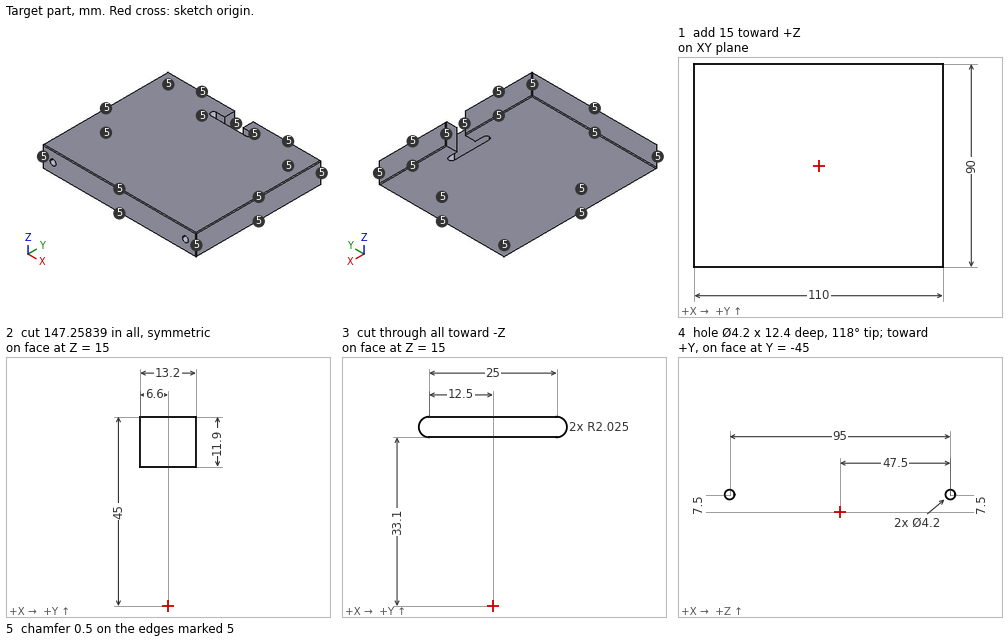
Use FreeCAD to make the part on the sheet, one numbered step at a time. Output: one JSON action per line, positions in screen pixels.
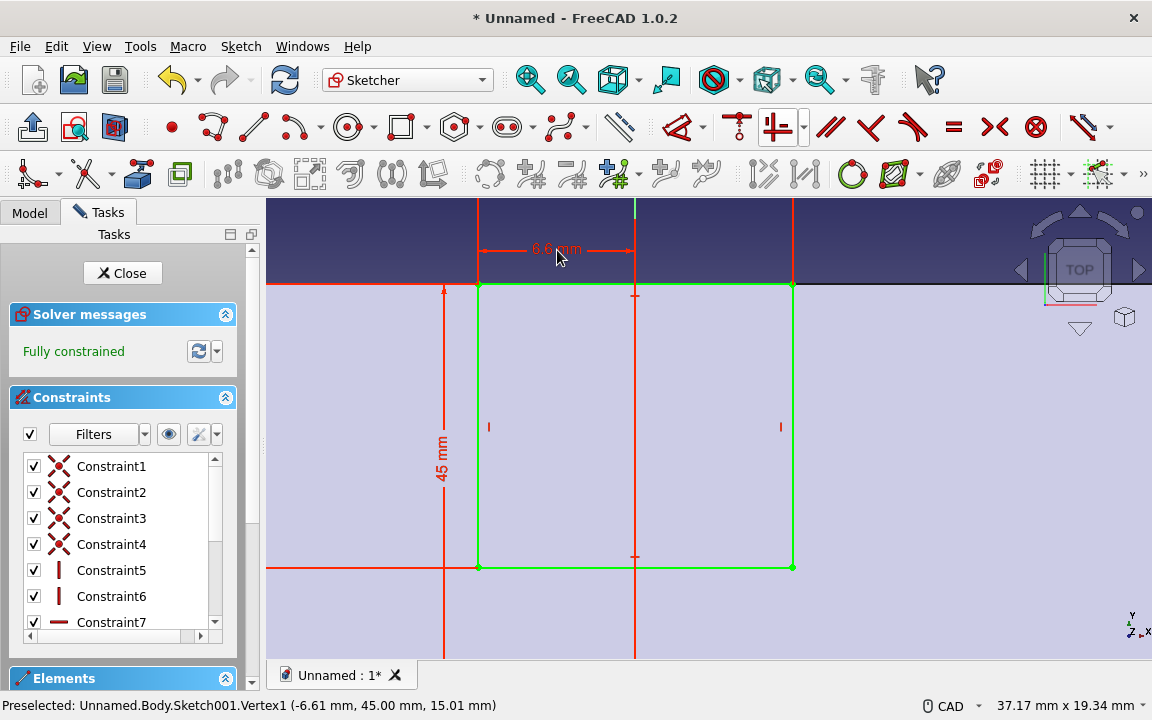
{"action": "left_click", "coordinate": [123, 273]}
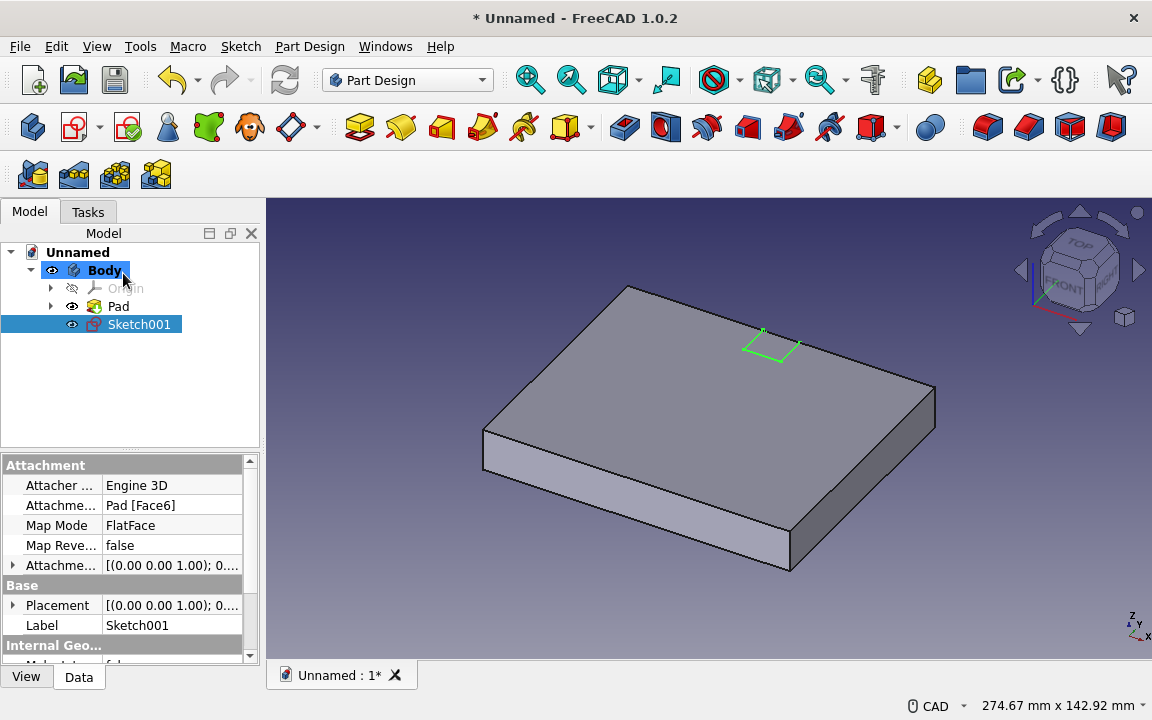
{"action": "left_click", "coordinate": [625, 128]}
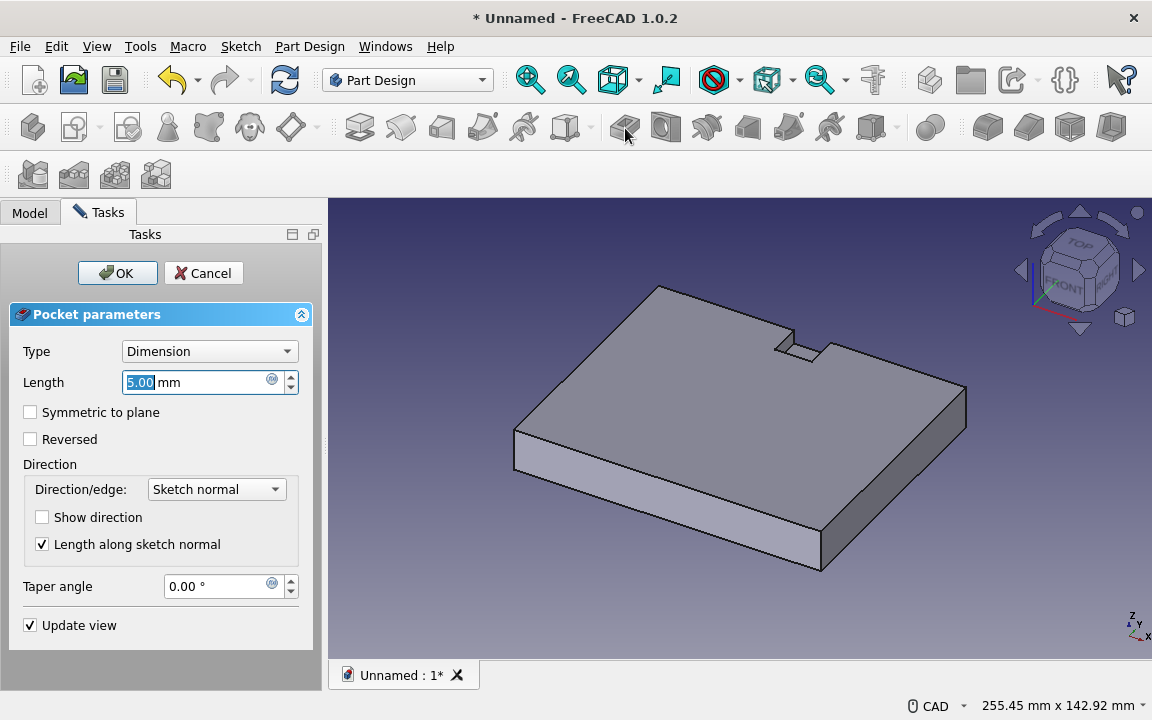
{"action": "type", "text": "147.25839"}
{"action": "key", "text": "Tab"}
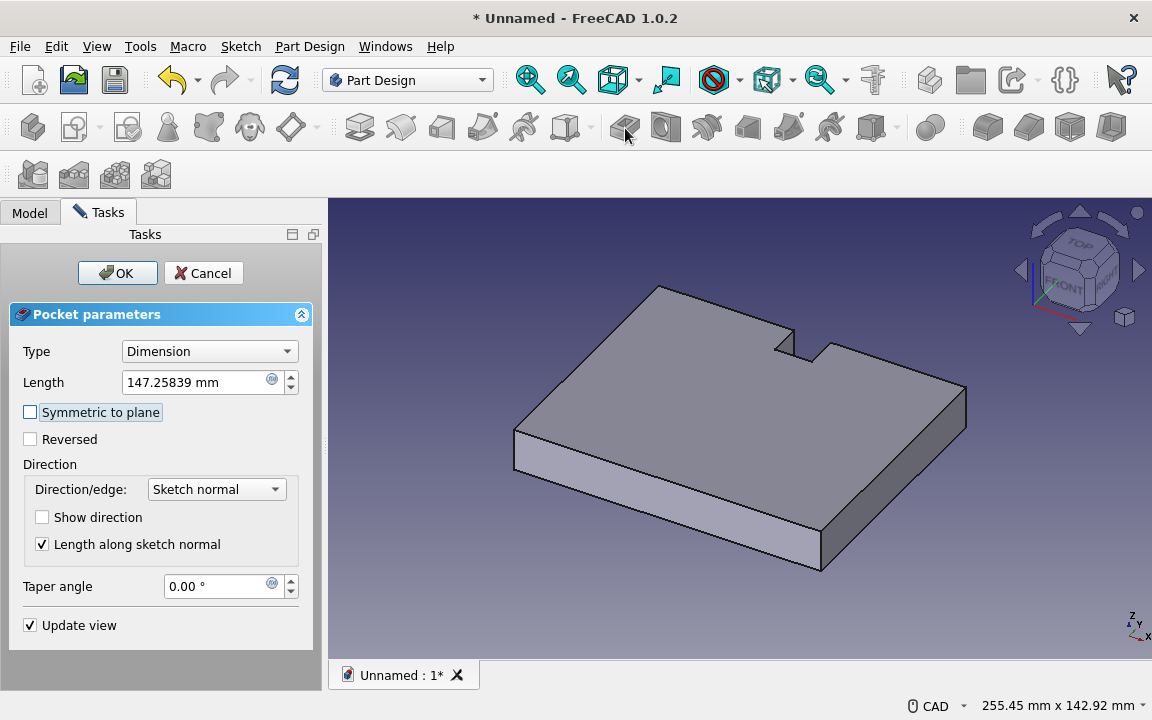
{"action": "left_click", "coordinate": [31, 412]}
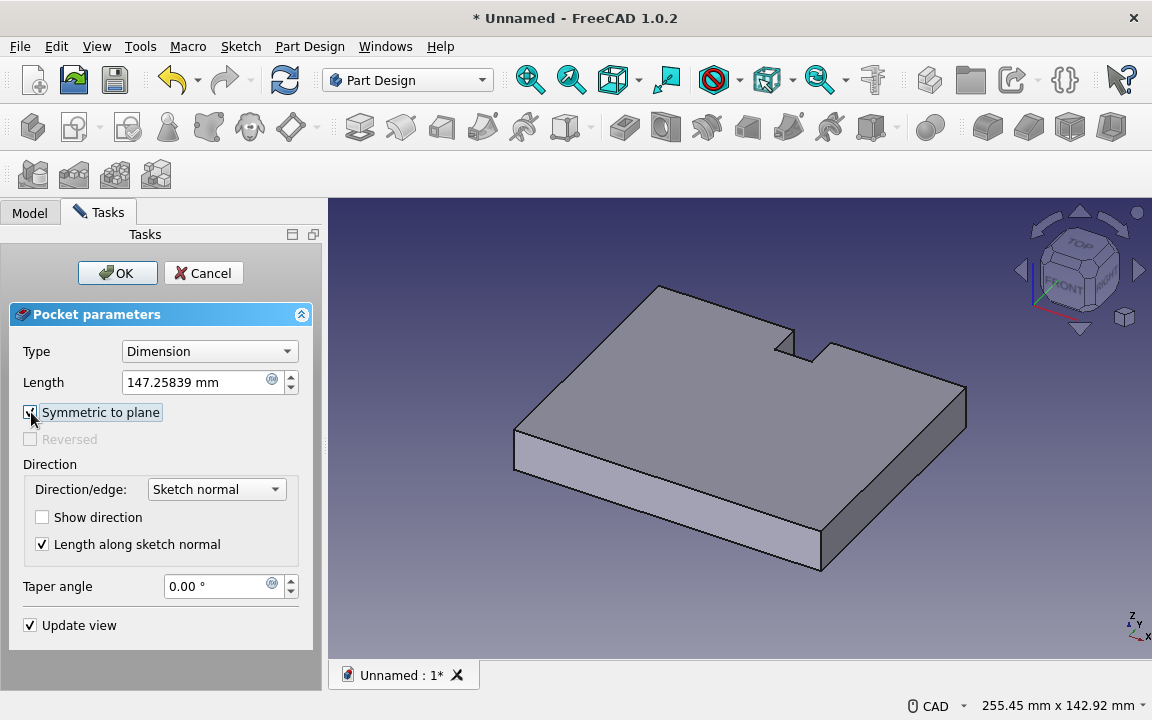
{"action": "left_click", "coordinate": [118, 273]}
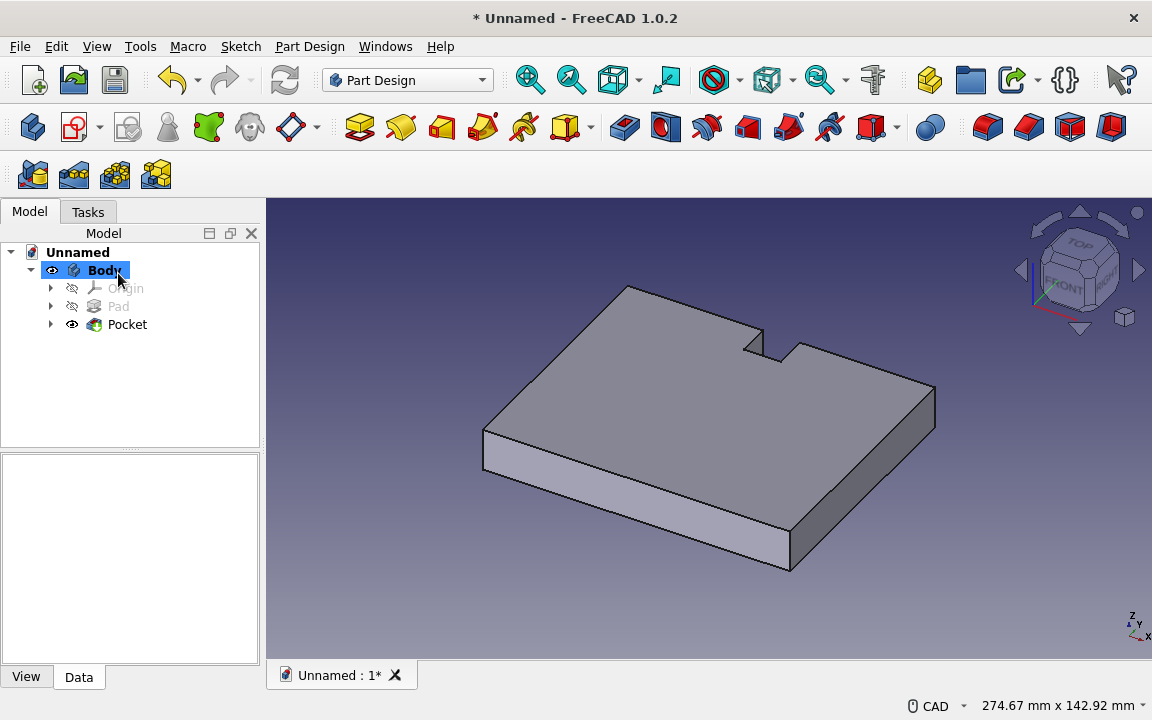
{"action": "left_click", "coordinate": [665, 393]}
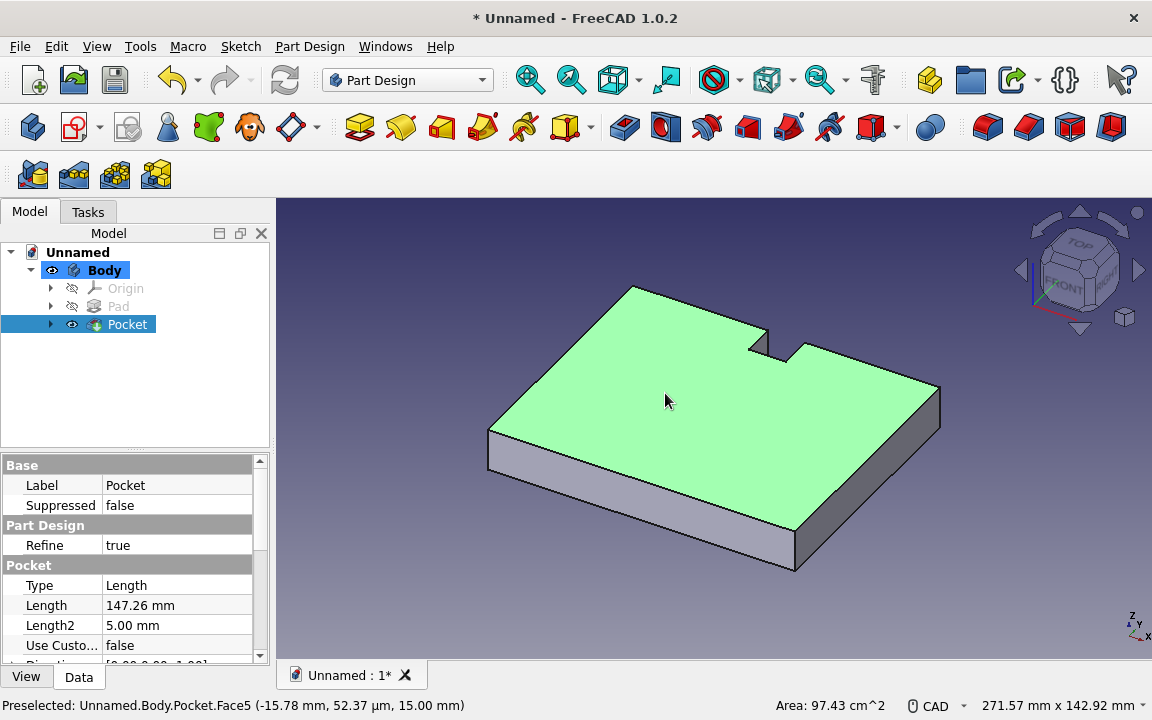
{"action": "left_click", "coordinate": [74, 128]}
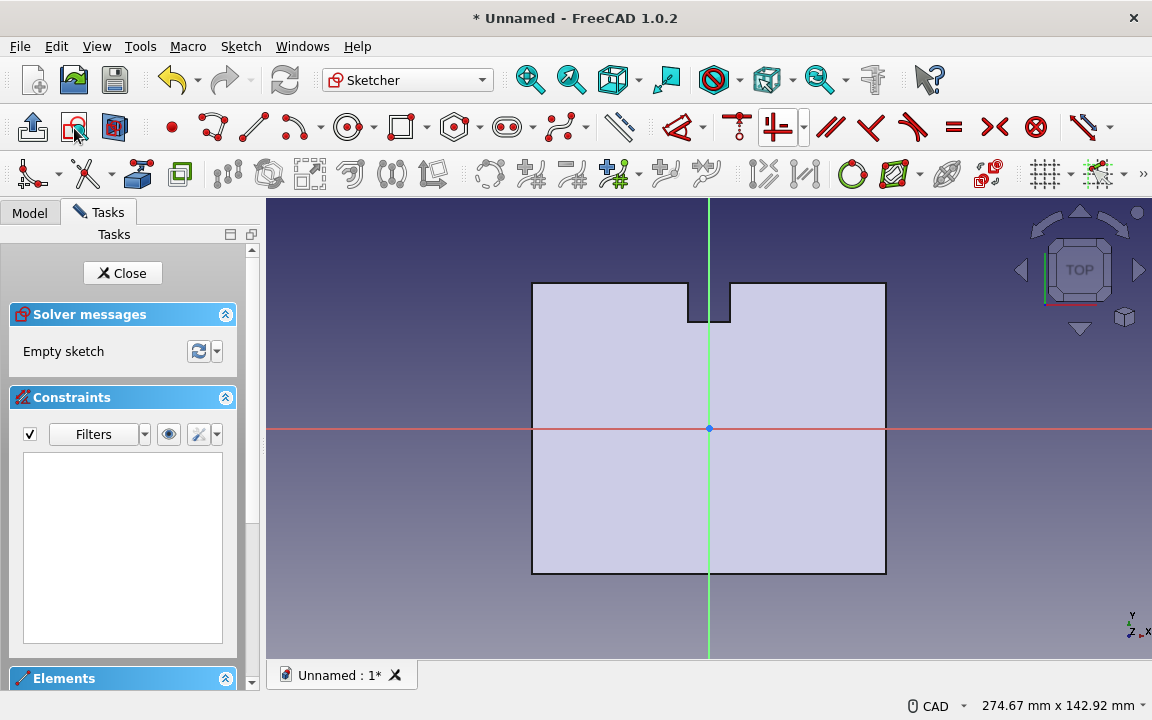
{"action": "scroll", "coordinate": [765, 320], "scroll_direction": "up", "scroll_amount": 4}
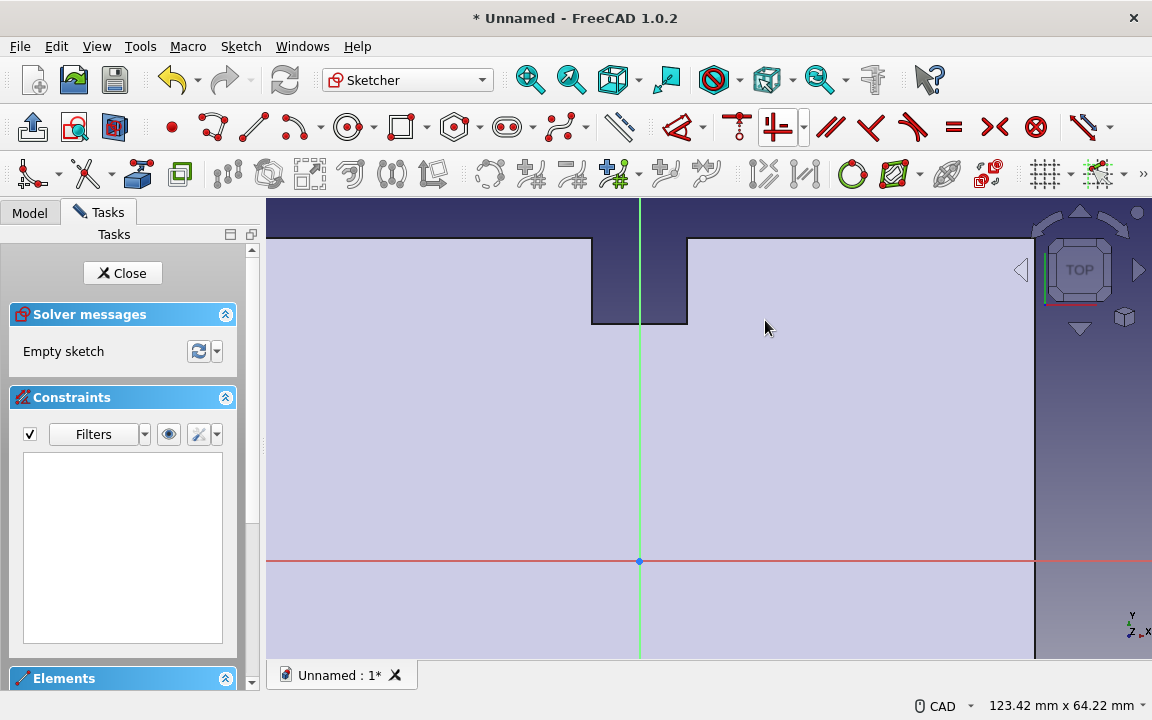
{"action": "left_click", "coordinate": [506, 128]}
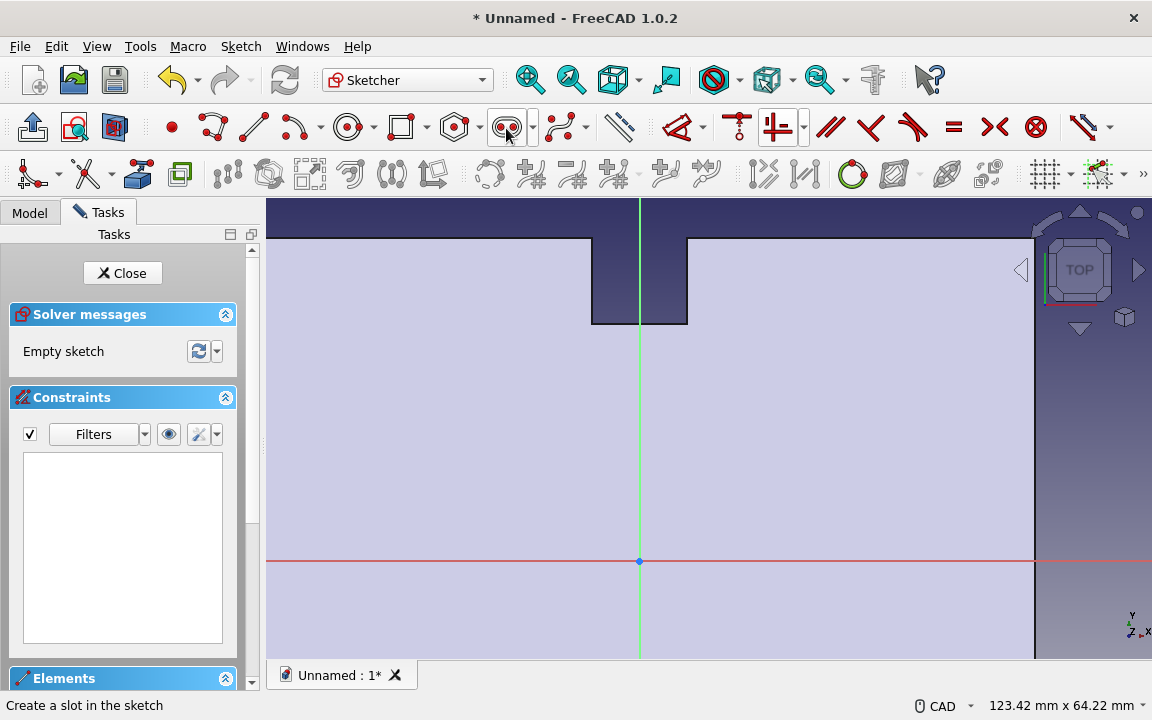
{"action": "scroll", "coordinate": [550, 309], "scroll_direction": "up", "scroll_amount": 3}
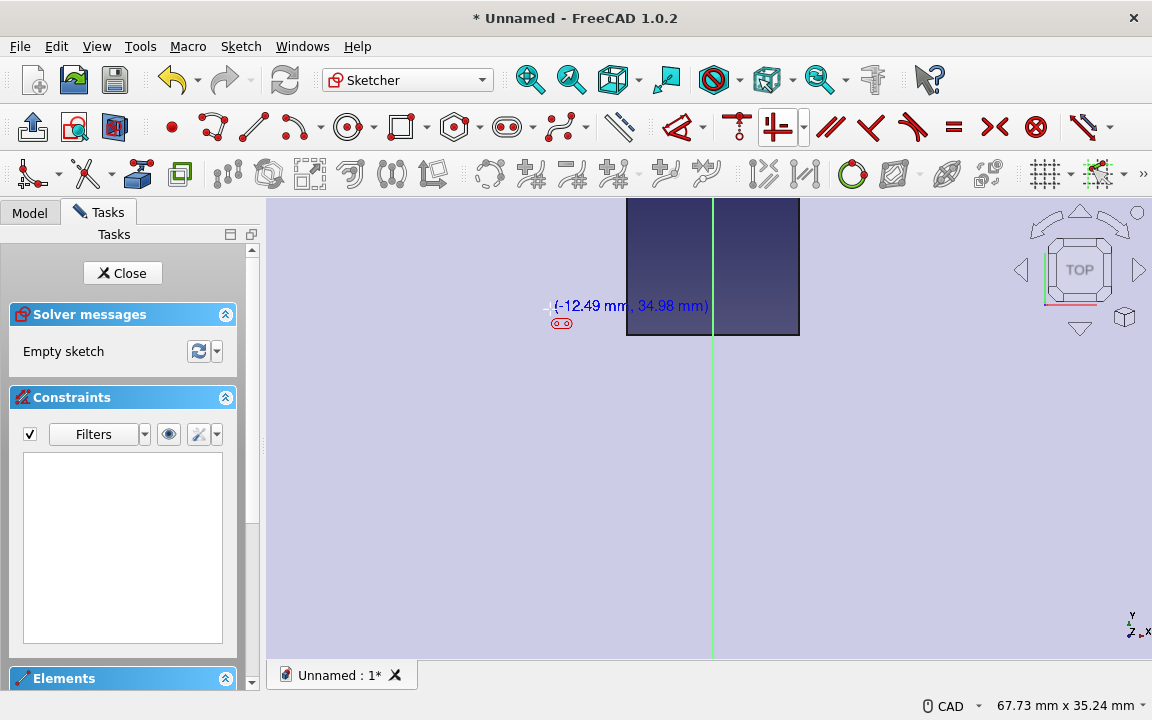
{"action": "left_click", "coordinate": [550, 309]}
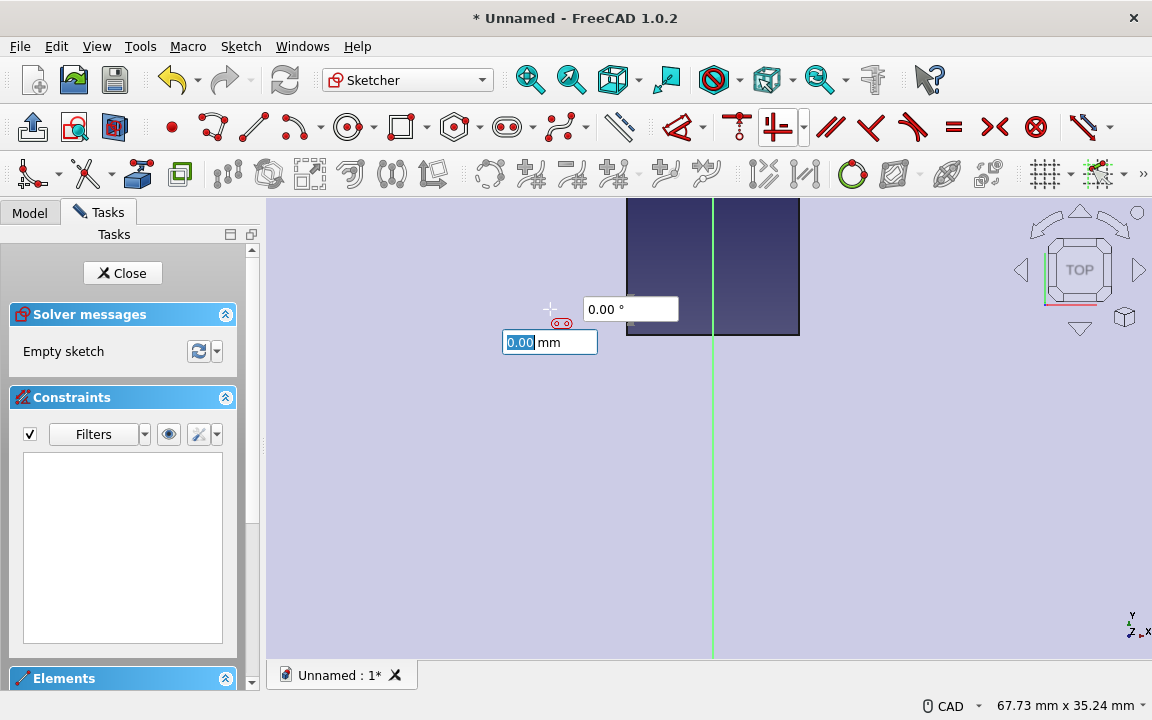
{"action": "left_click", "coordinate": [877, 309]}